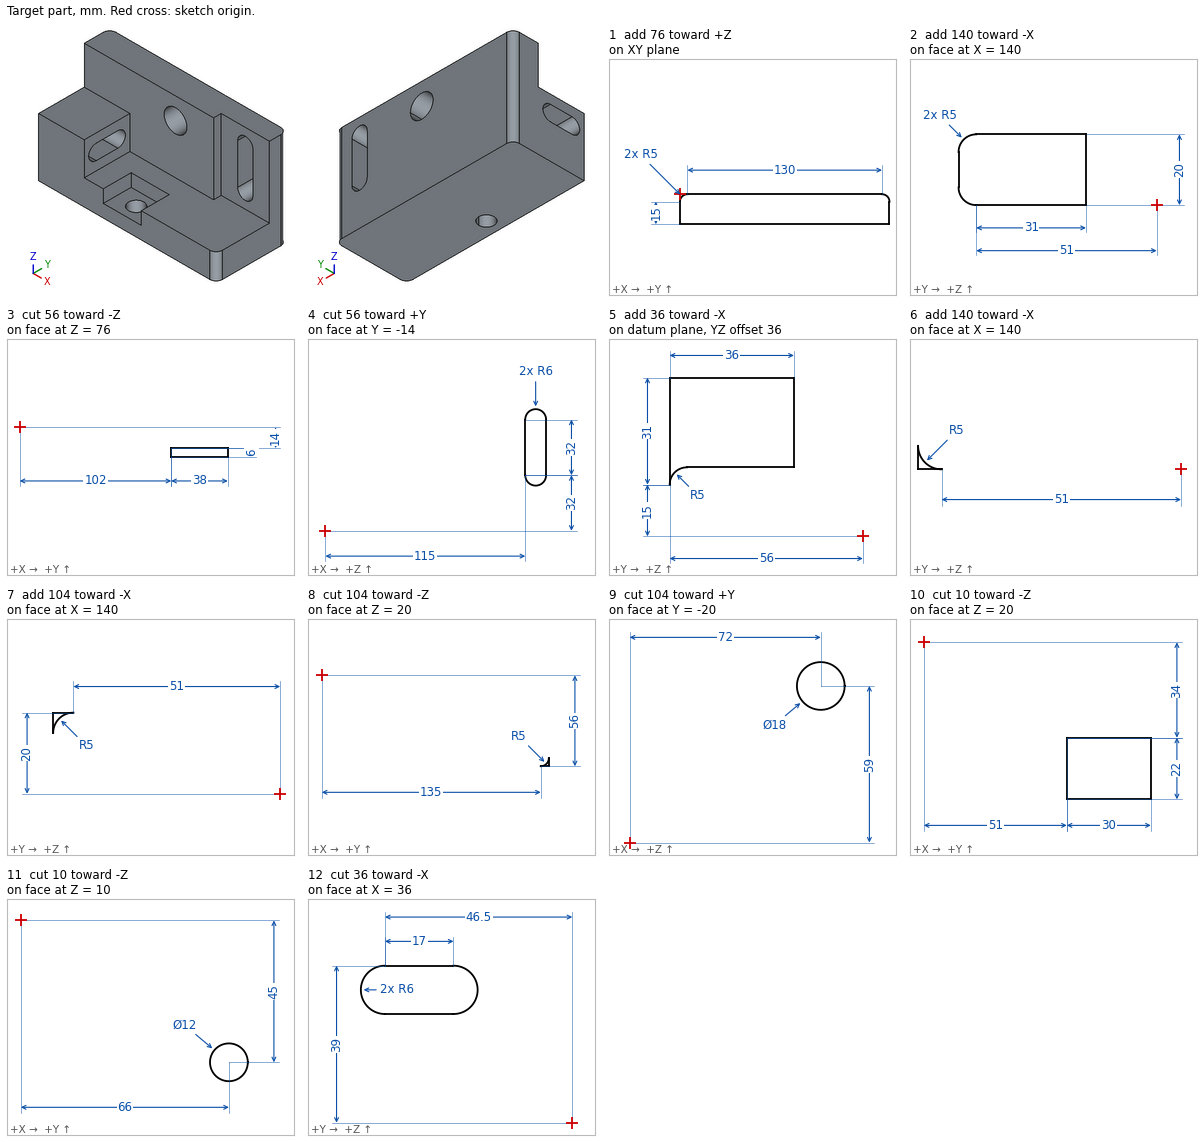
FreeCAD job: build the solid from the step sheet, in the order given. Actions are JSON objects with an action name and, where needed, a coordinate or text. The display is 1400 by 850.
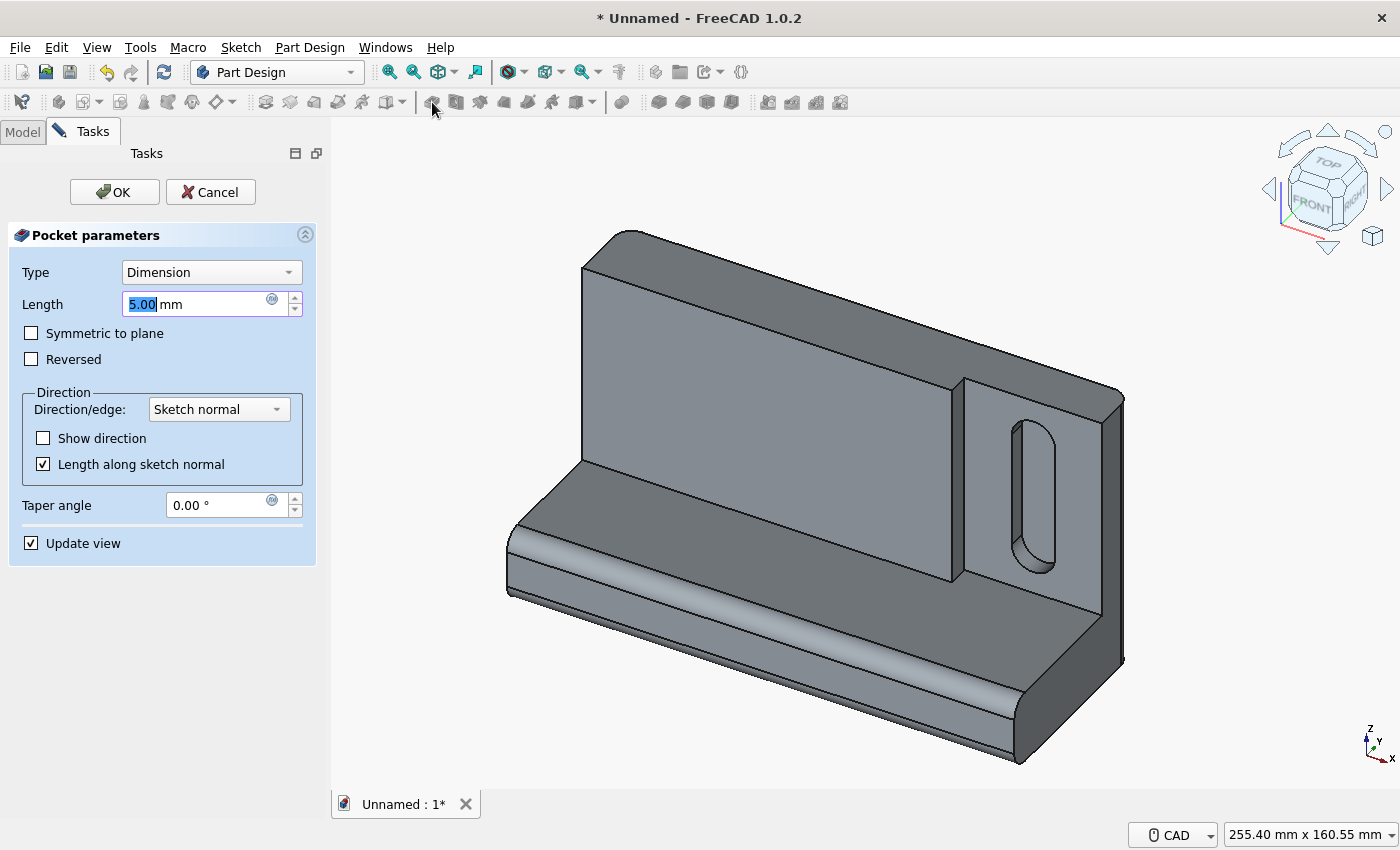
{"action": "type", "text": "56"}
{"action": "key", "text": "Tab"}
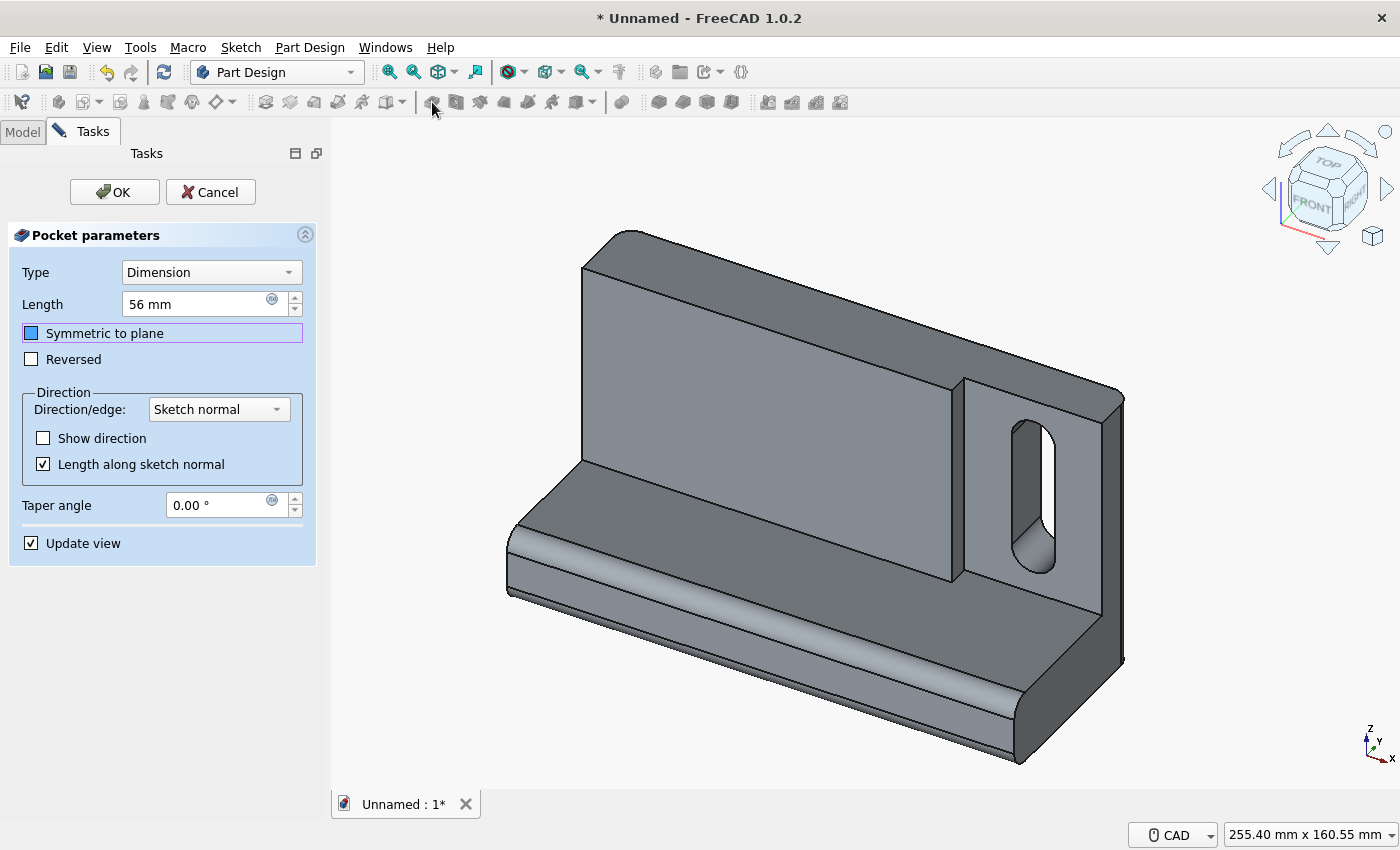
{"action": "left_click", "coordinate": [115, 192]}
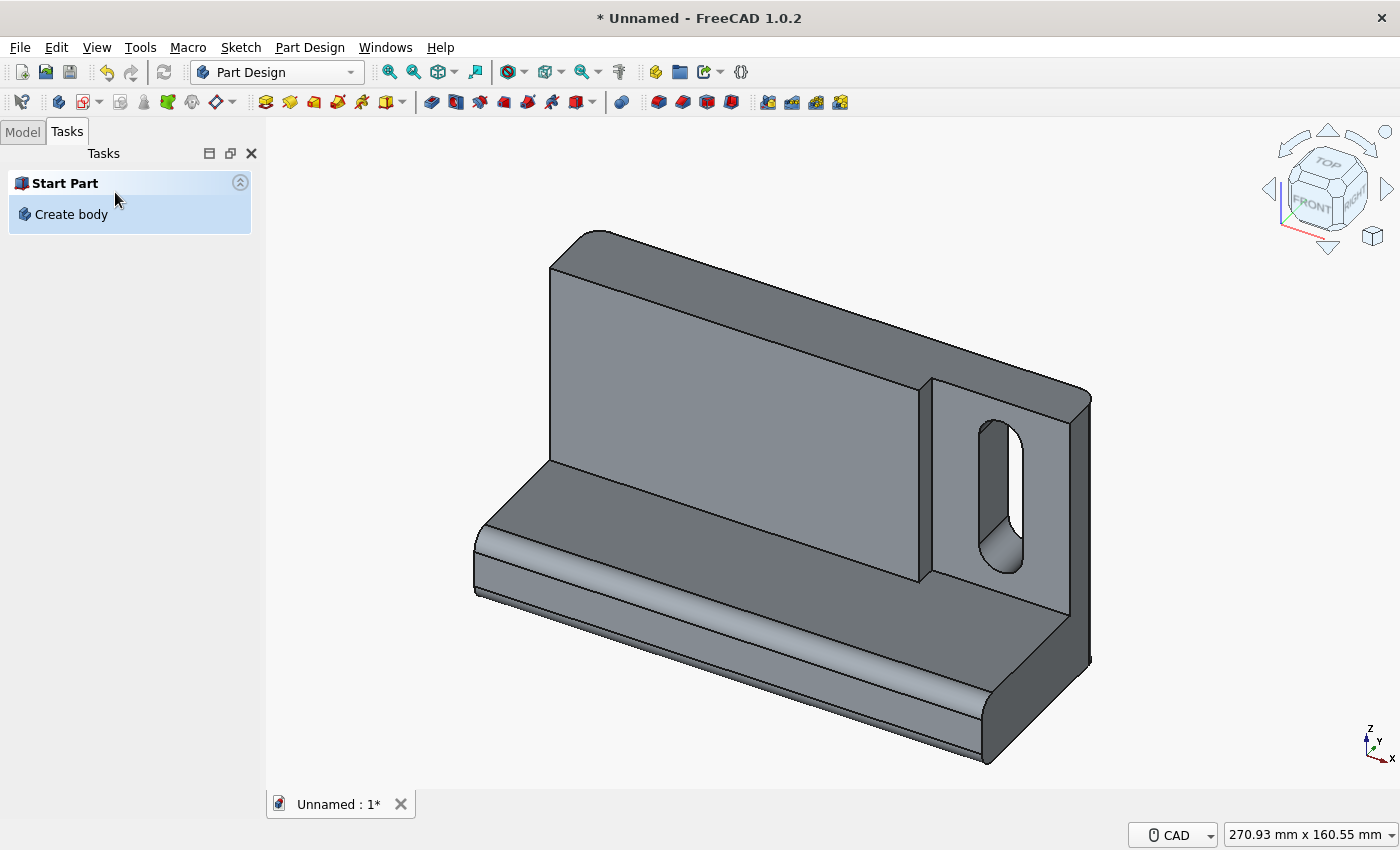
{"action": "left_click", "coordinate": [23, 131]}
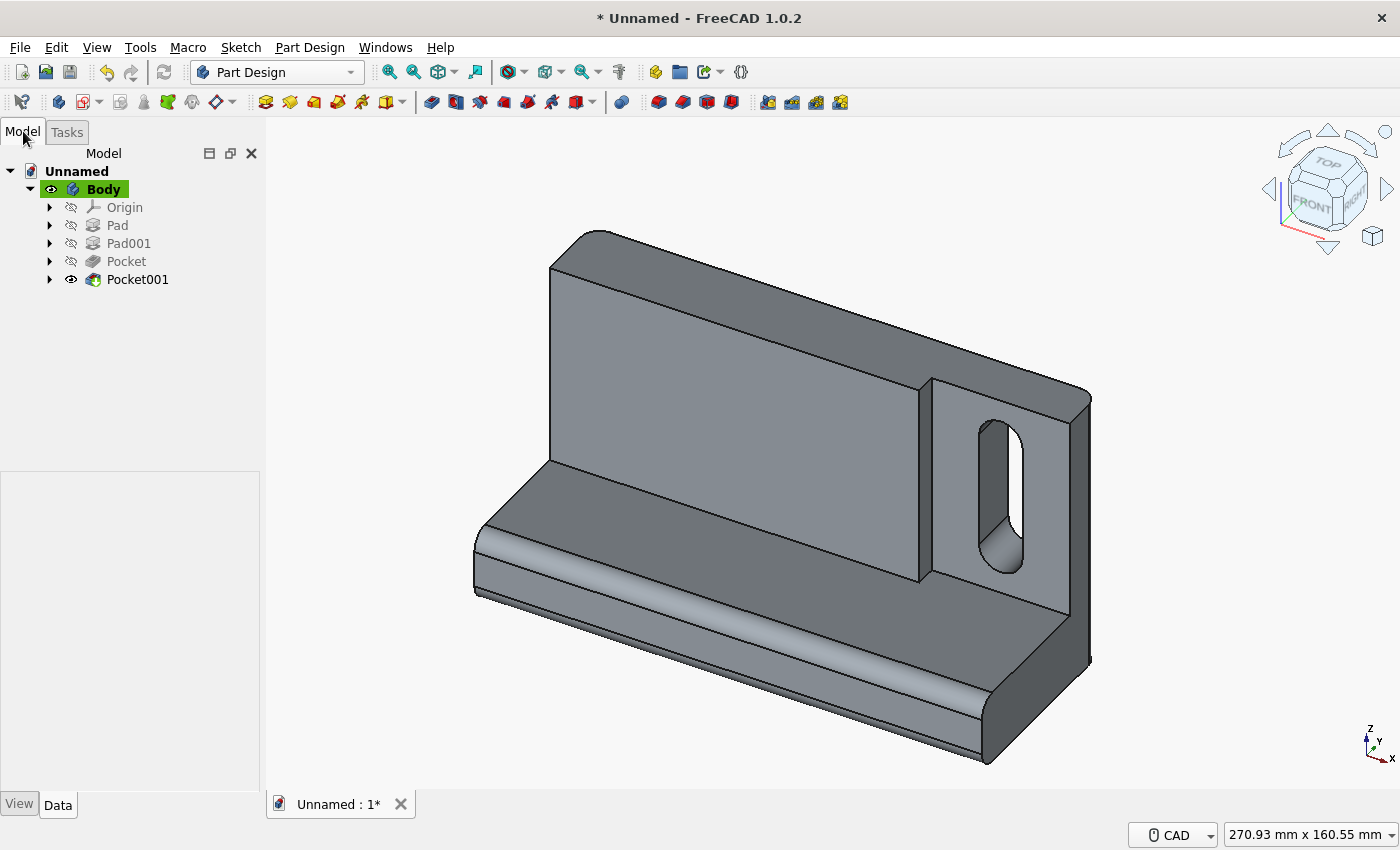
{"action": "left_click", "coordinate": [50, 207]}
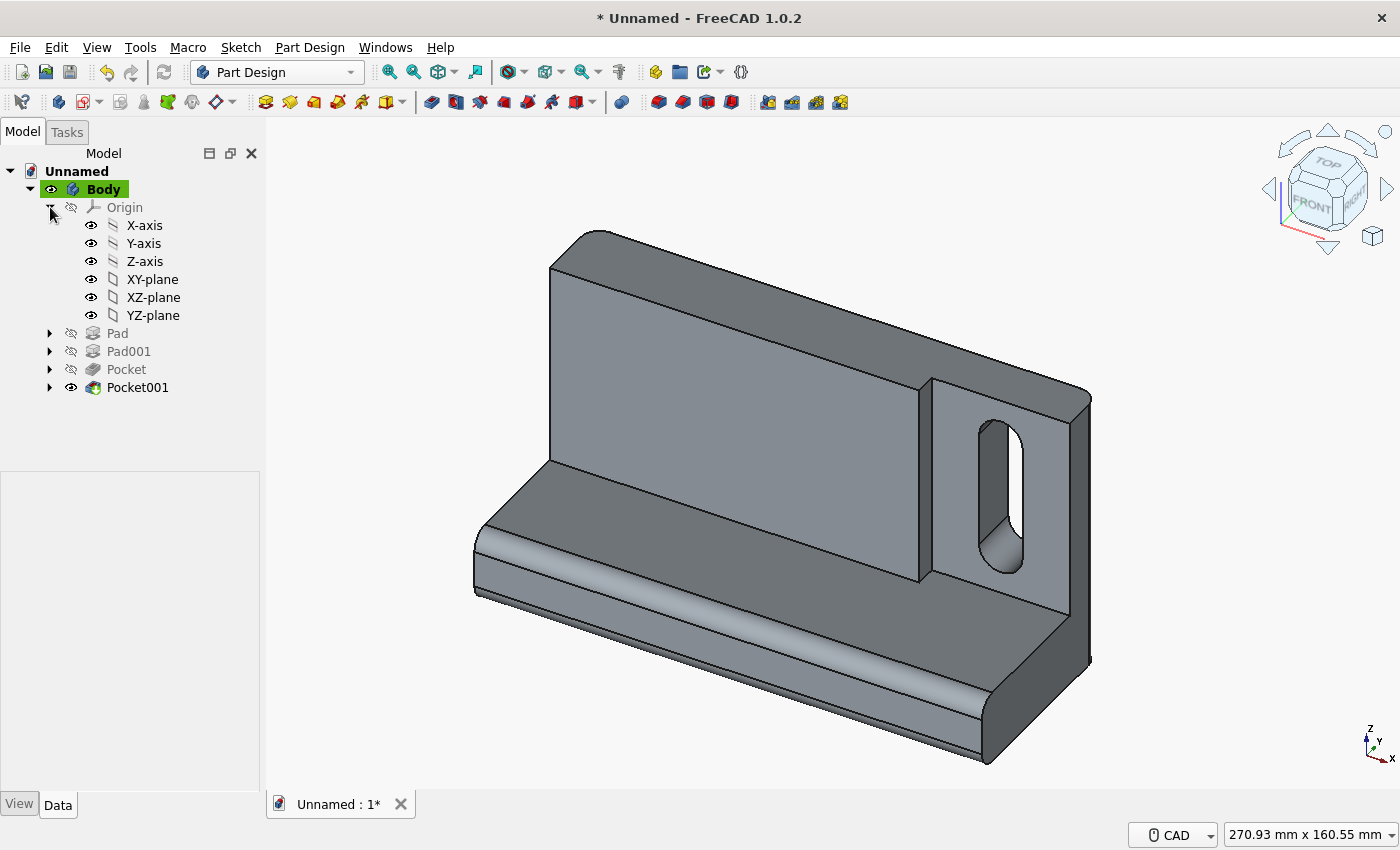
{"action": "left_click", "coordinate": [136, 315]}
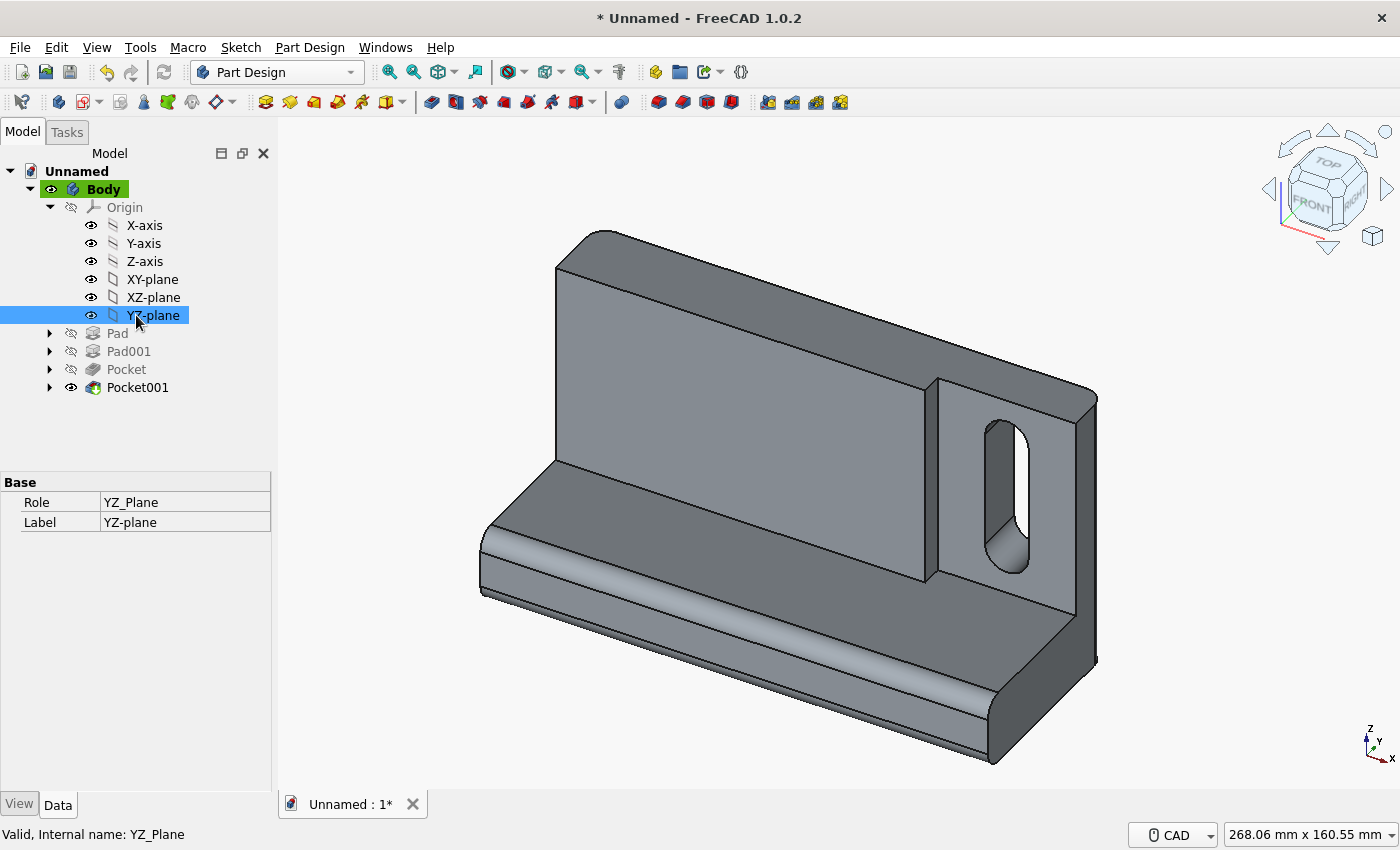
{"action": "left_click", "coordinate": [216, 102]}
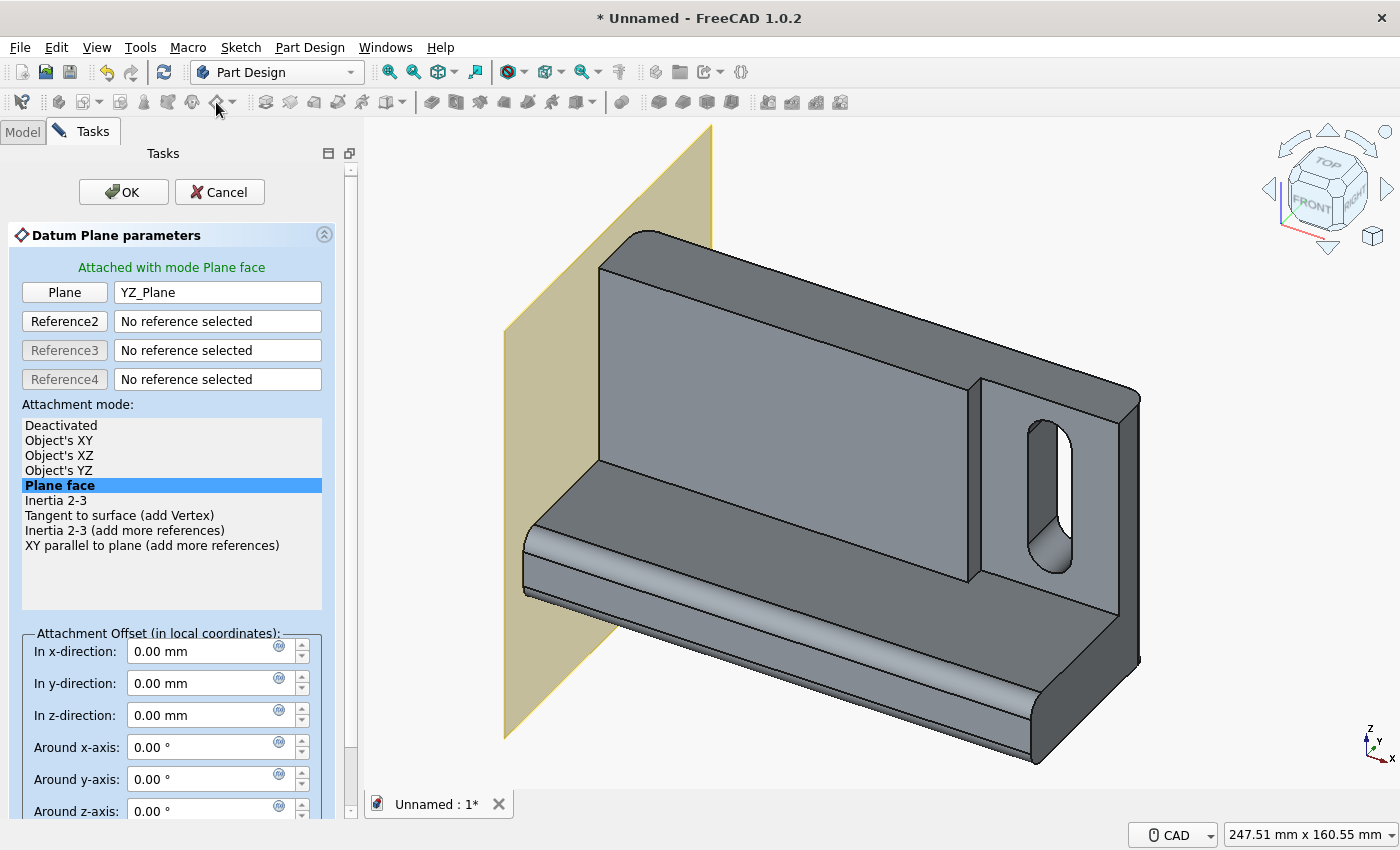
{"action": "triple_click", "coordinate": [210, 715]}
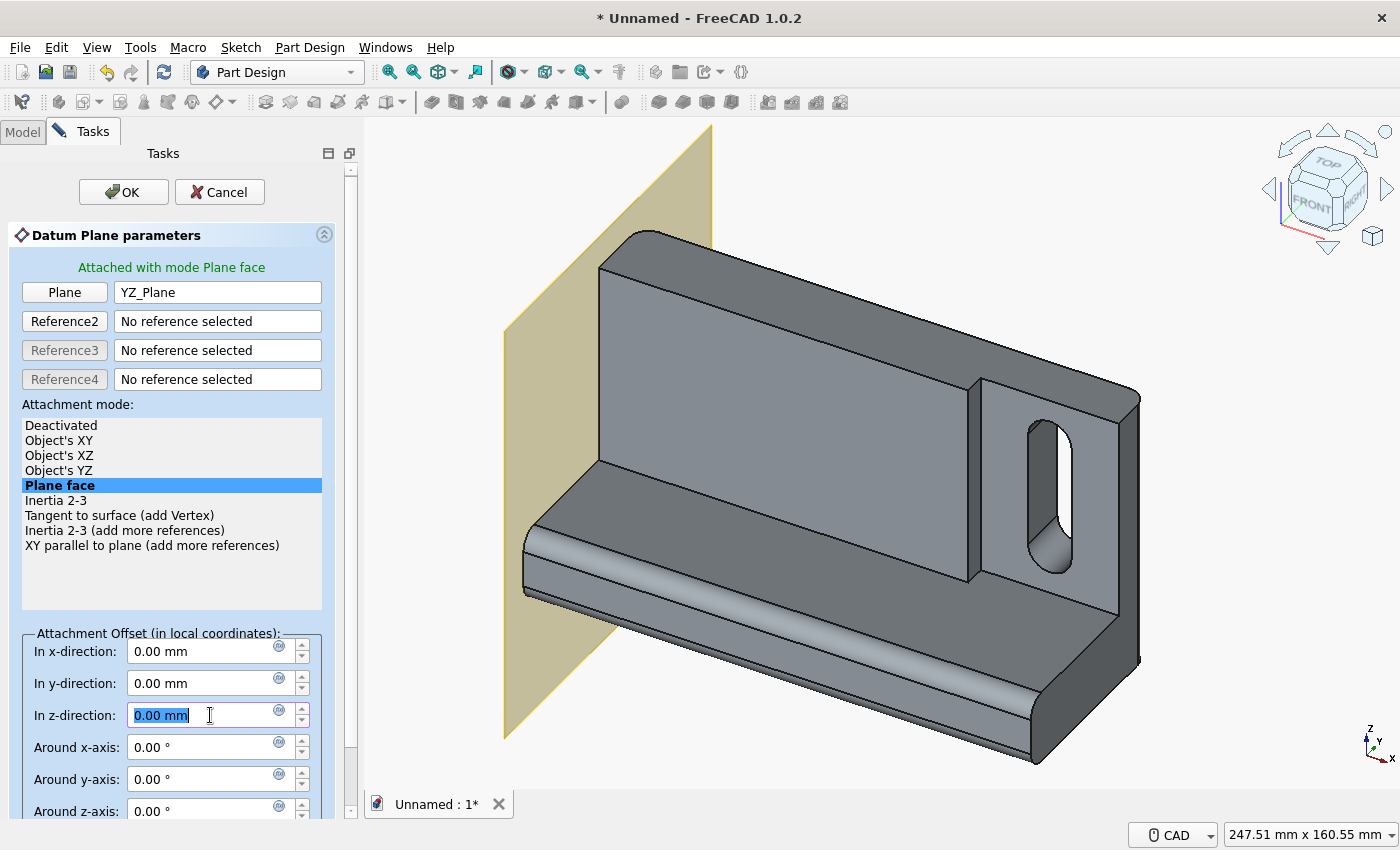
{"action": "type", "text": "36"}
{"action": "key", "text": "Tab"}